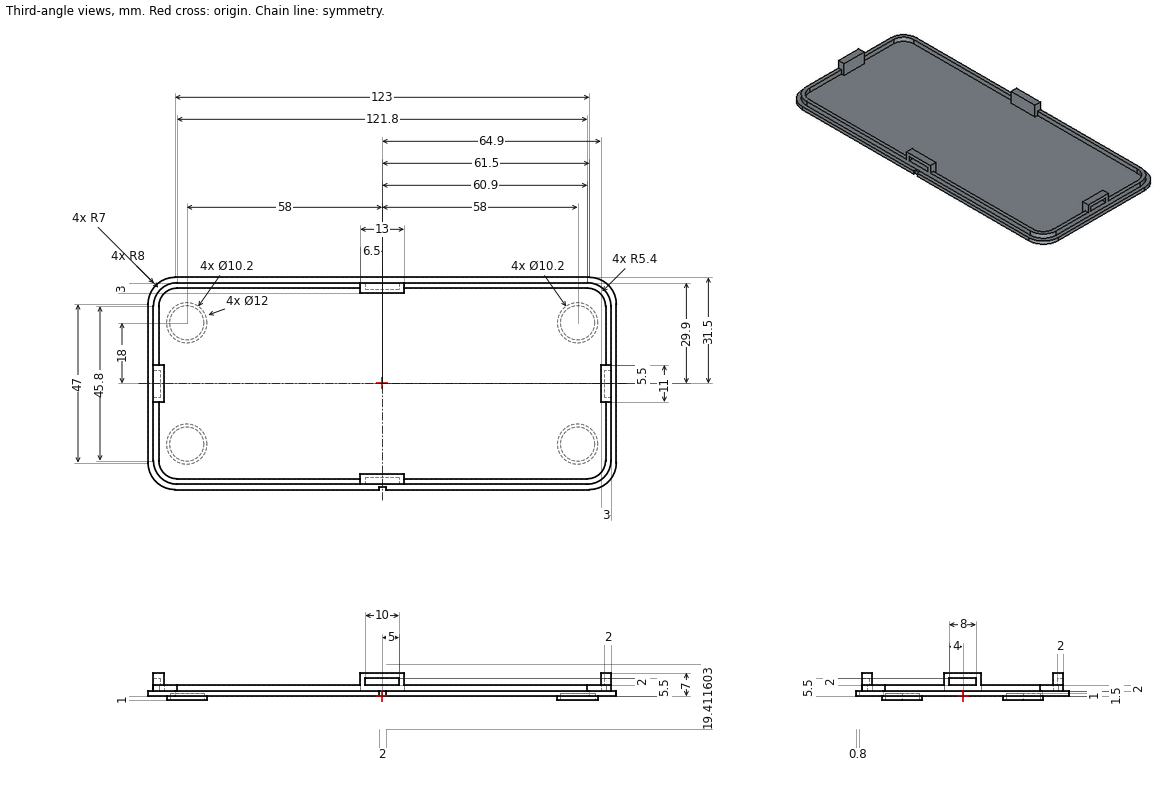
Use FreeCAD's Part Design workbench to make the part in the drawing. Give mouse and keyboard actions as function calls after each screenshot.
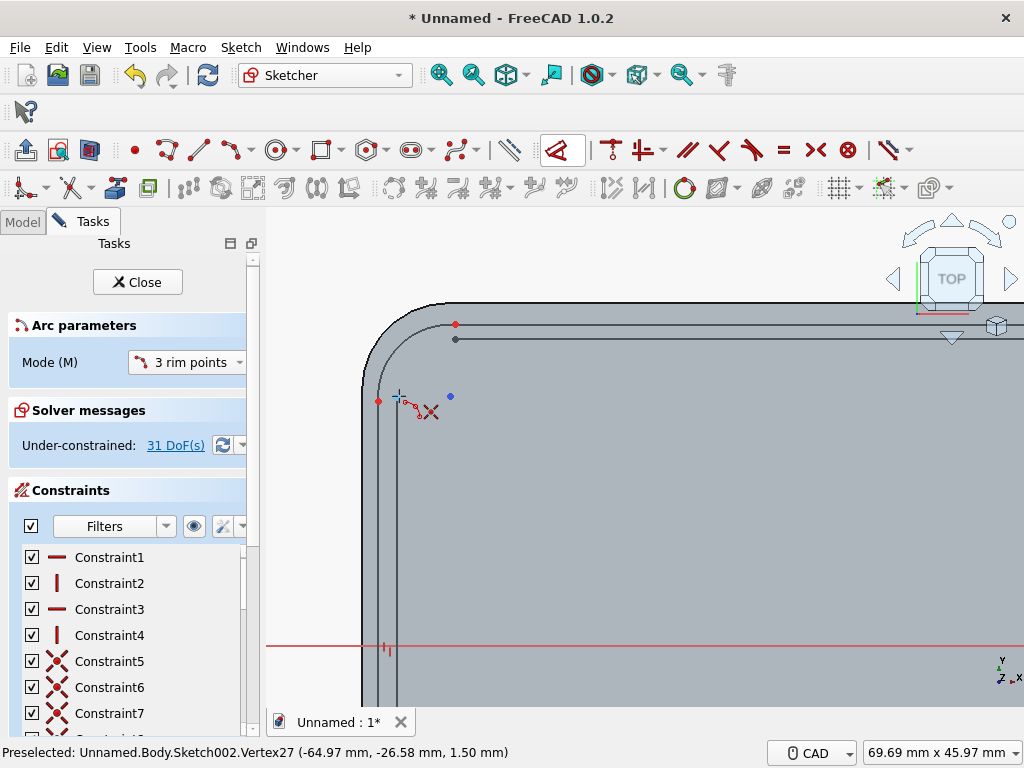
click(397, 398)
click(456, 339)
click(414, 355)
key(Escape)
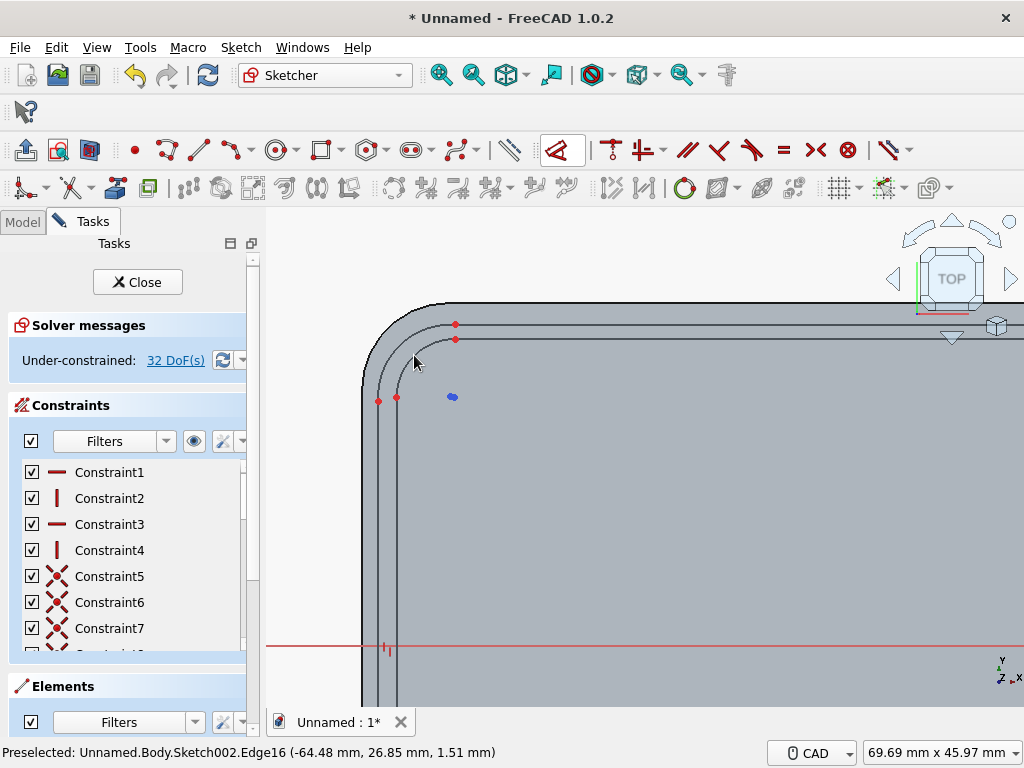
click(853, 325)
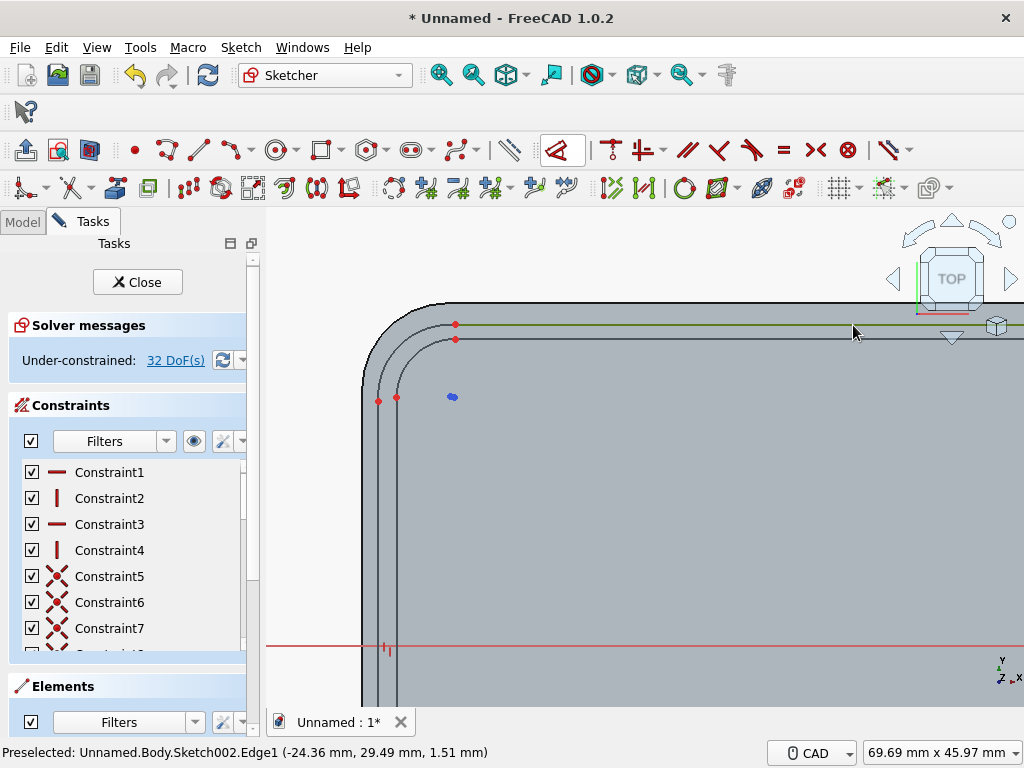
click(419, 332)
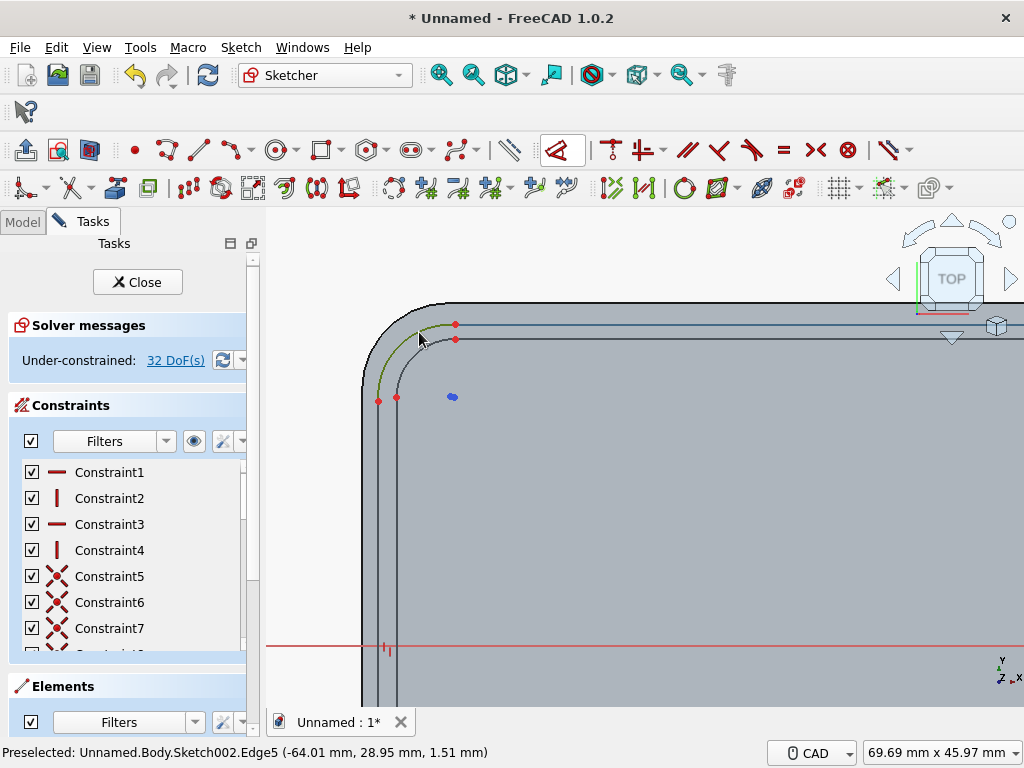
key(t)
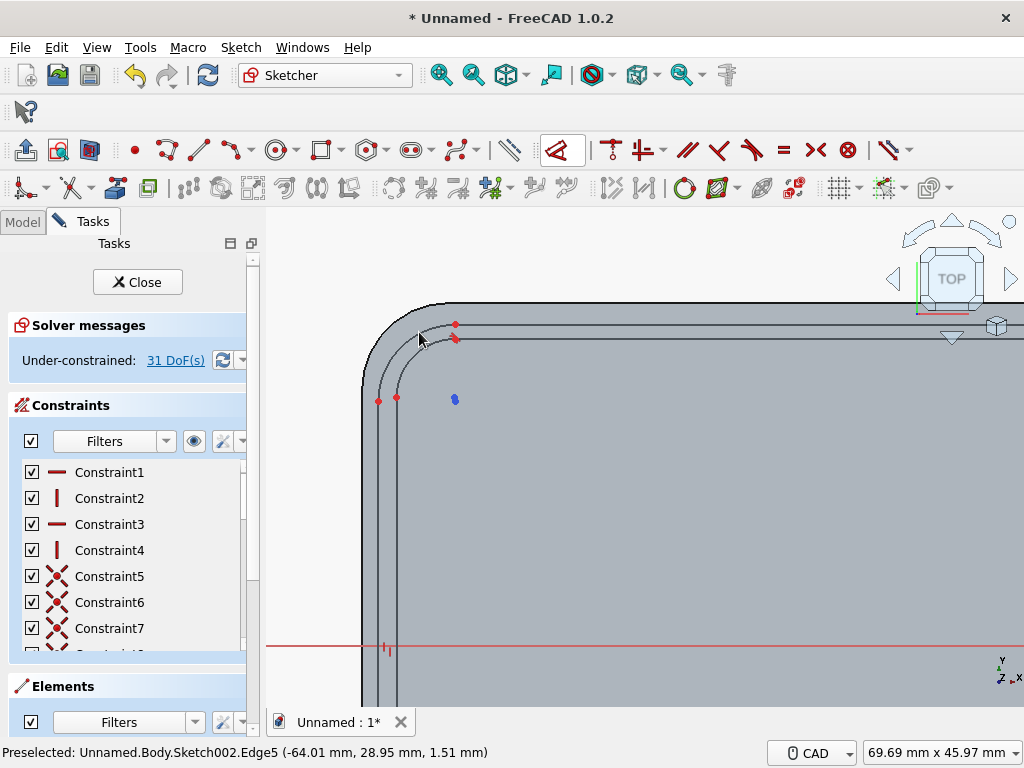
click(853, 325)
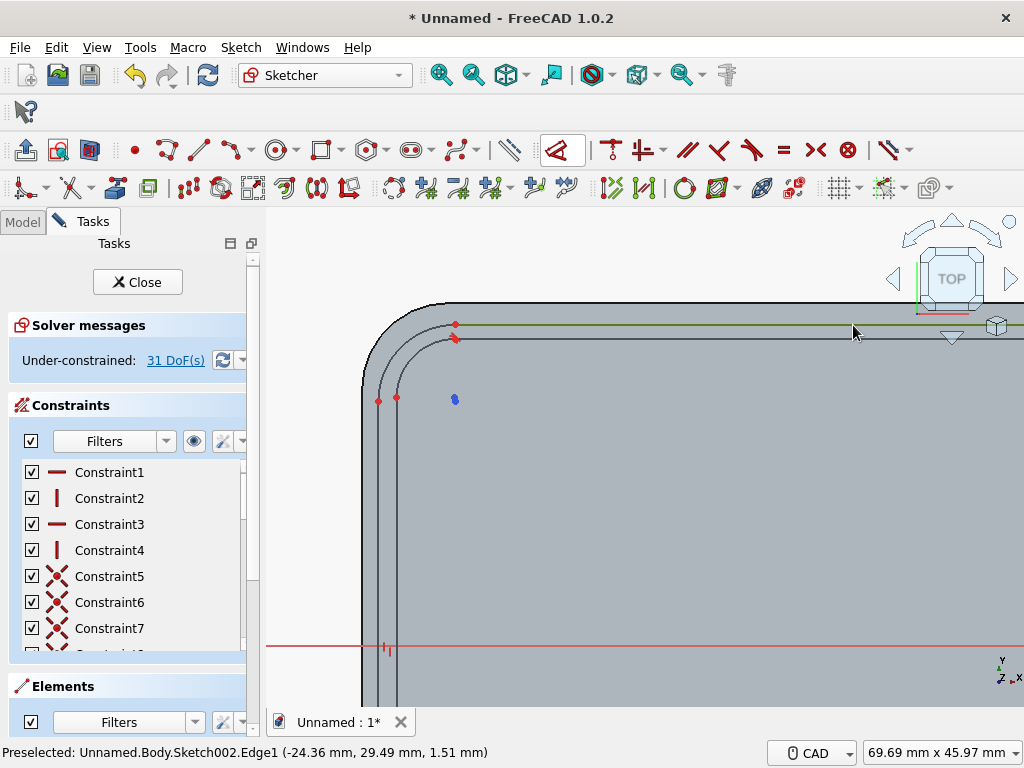
scroll(399, 395, down, 7)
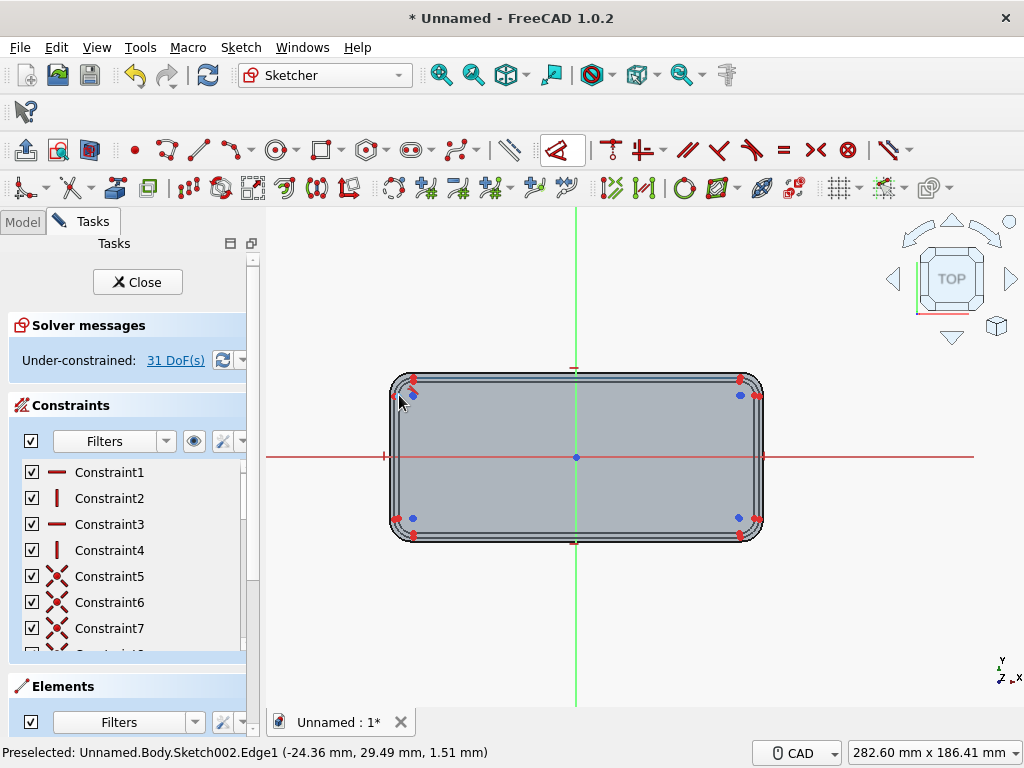
scroll(757, 388, up, 6)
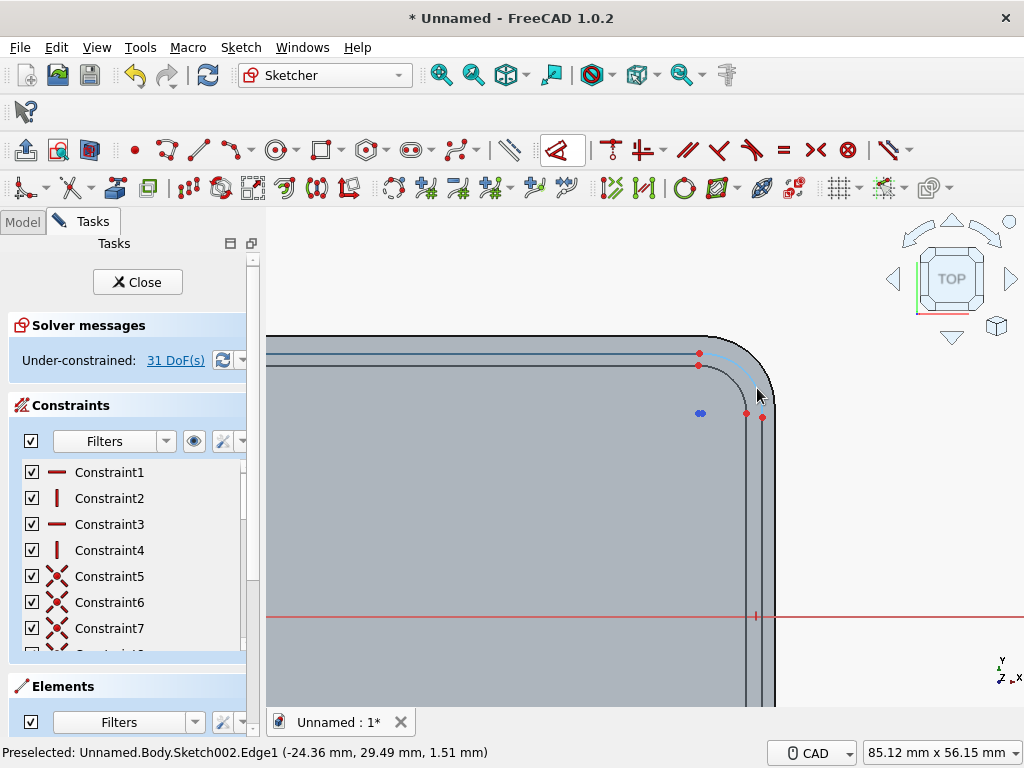
click(757, 388)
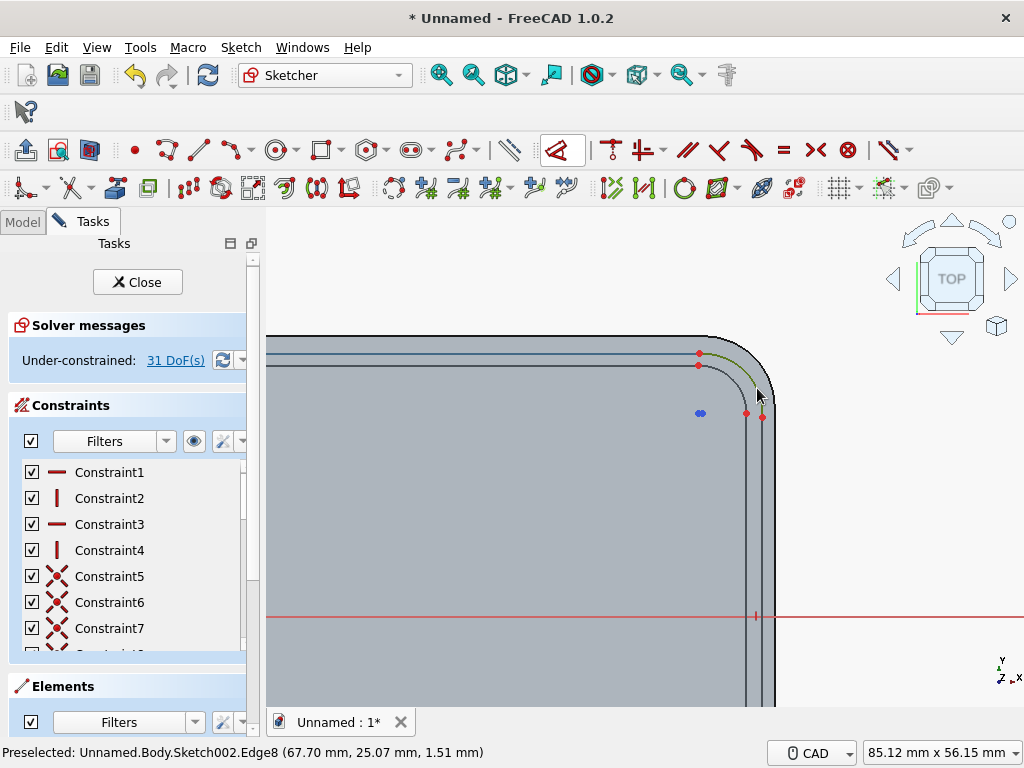
key(t)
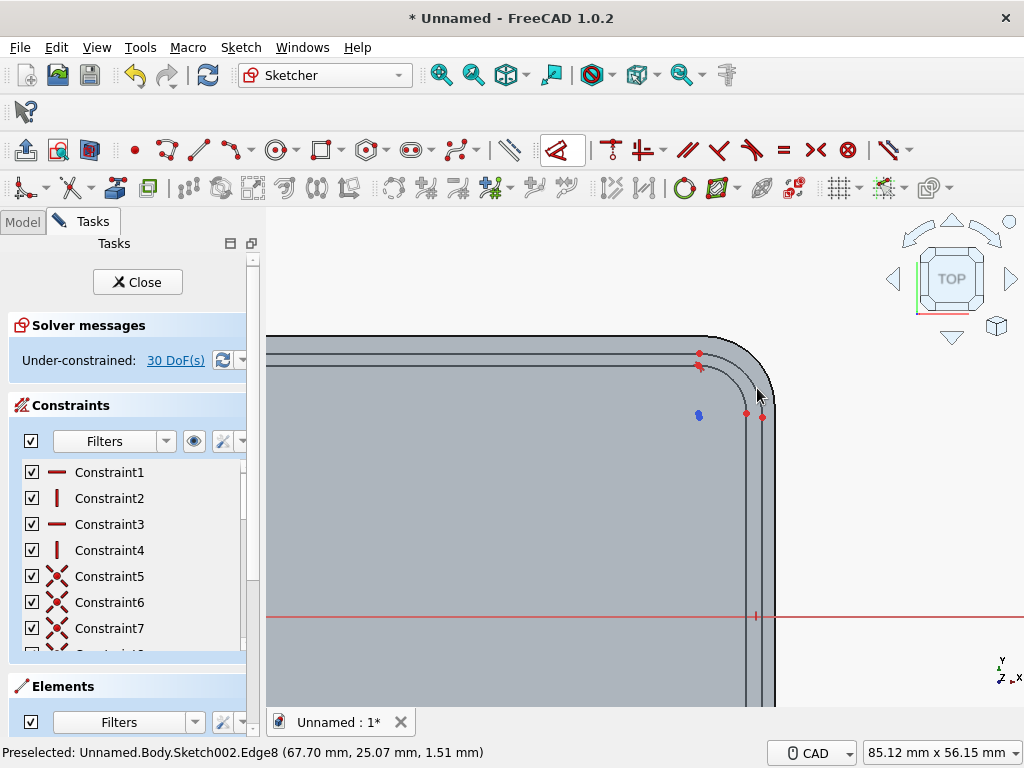
scroll(758, 388, down, 6)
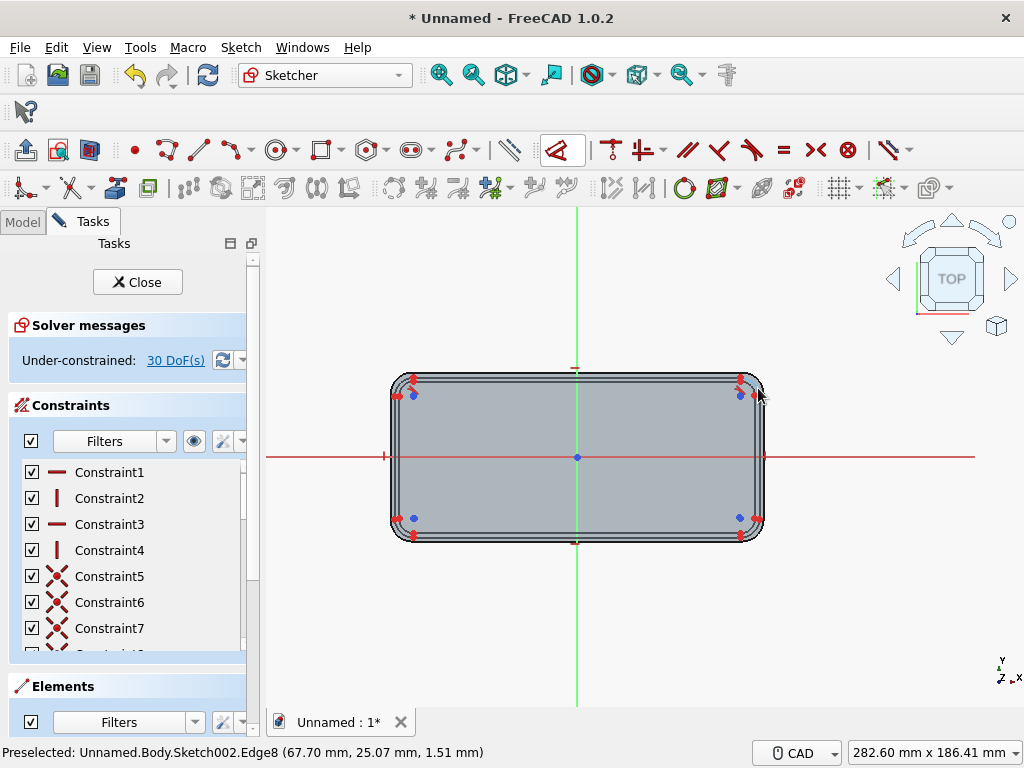
scroll(395, 434, up, 6)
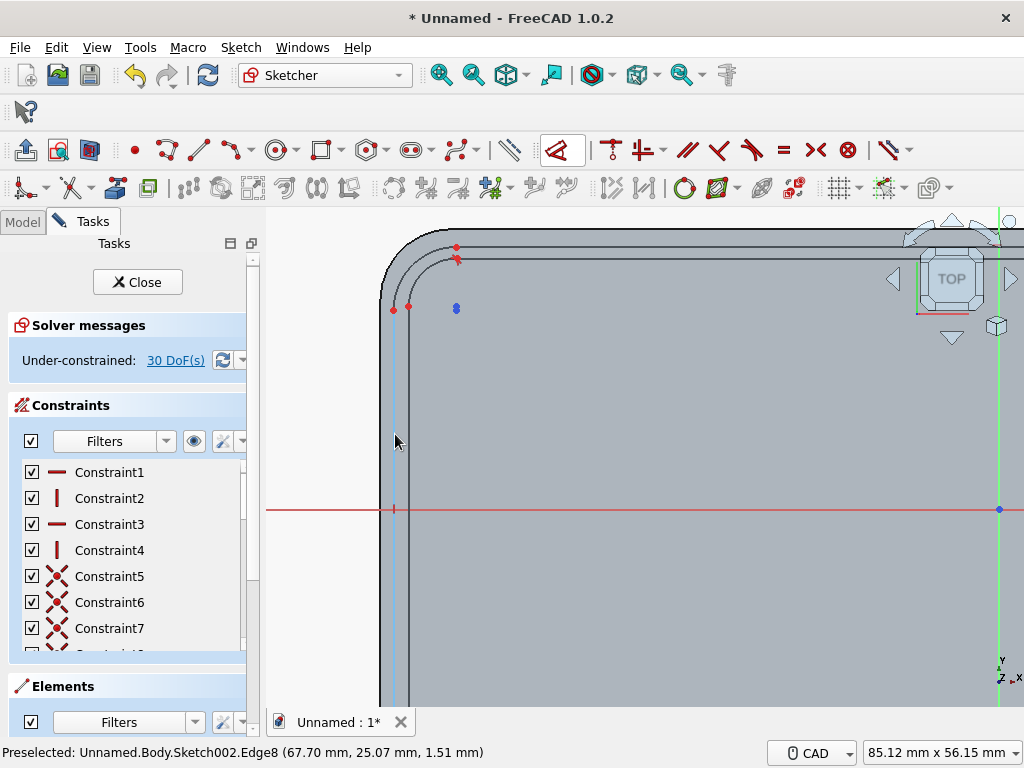
click(394, 433)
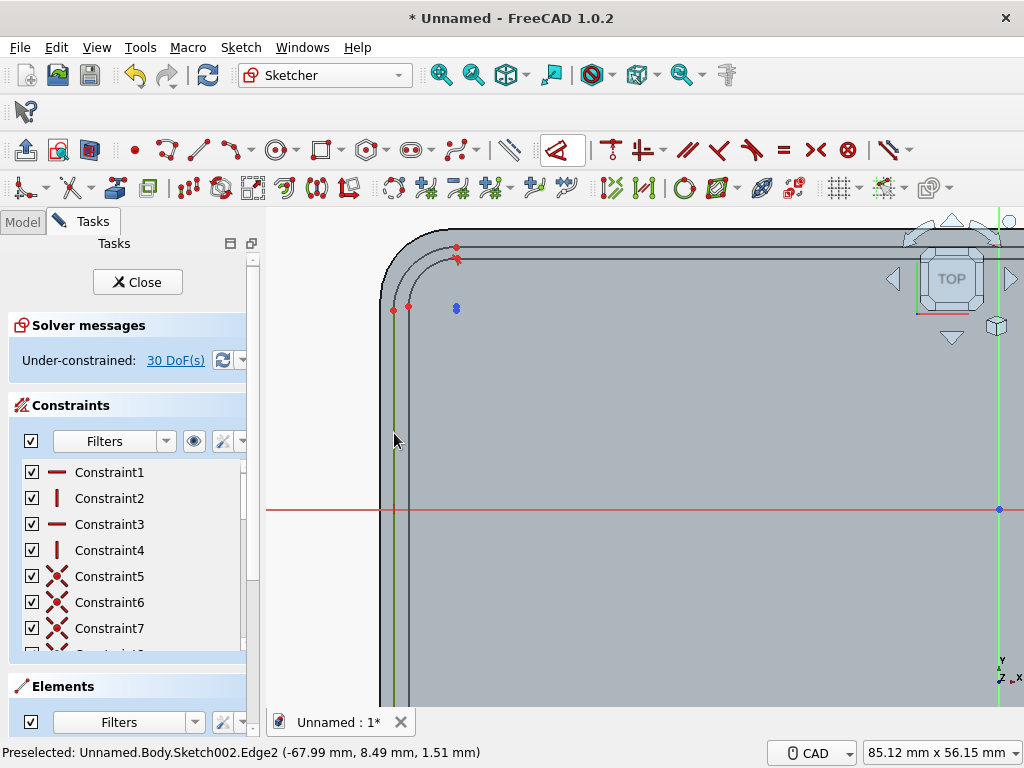
click(428, 254)